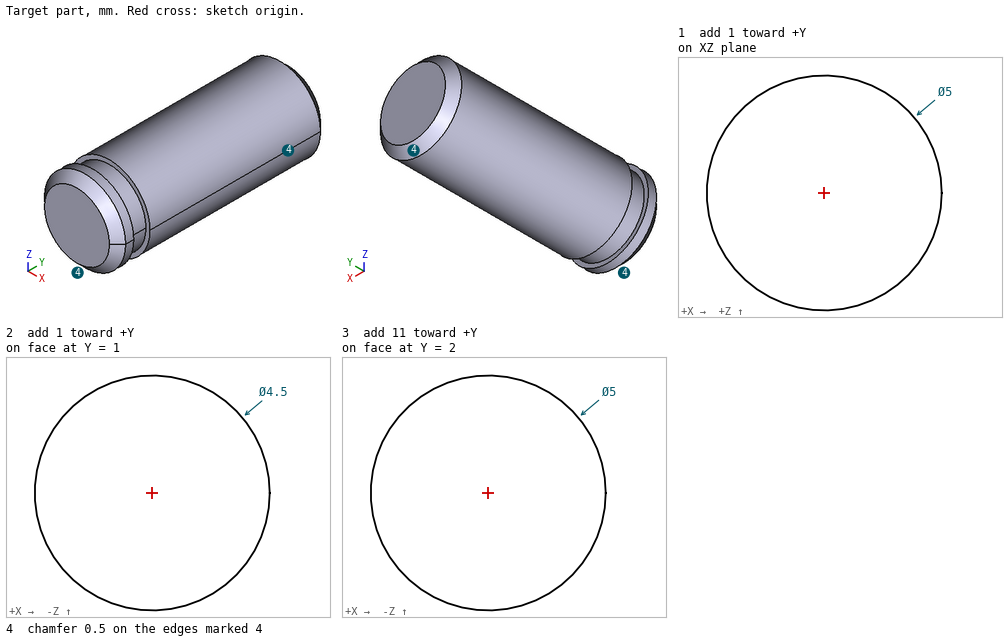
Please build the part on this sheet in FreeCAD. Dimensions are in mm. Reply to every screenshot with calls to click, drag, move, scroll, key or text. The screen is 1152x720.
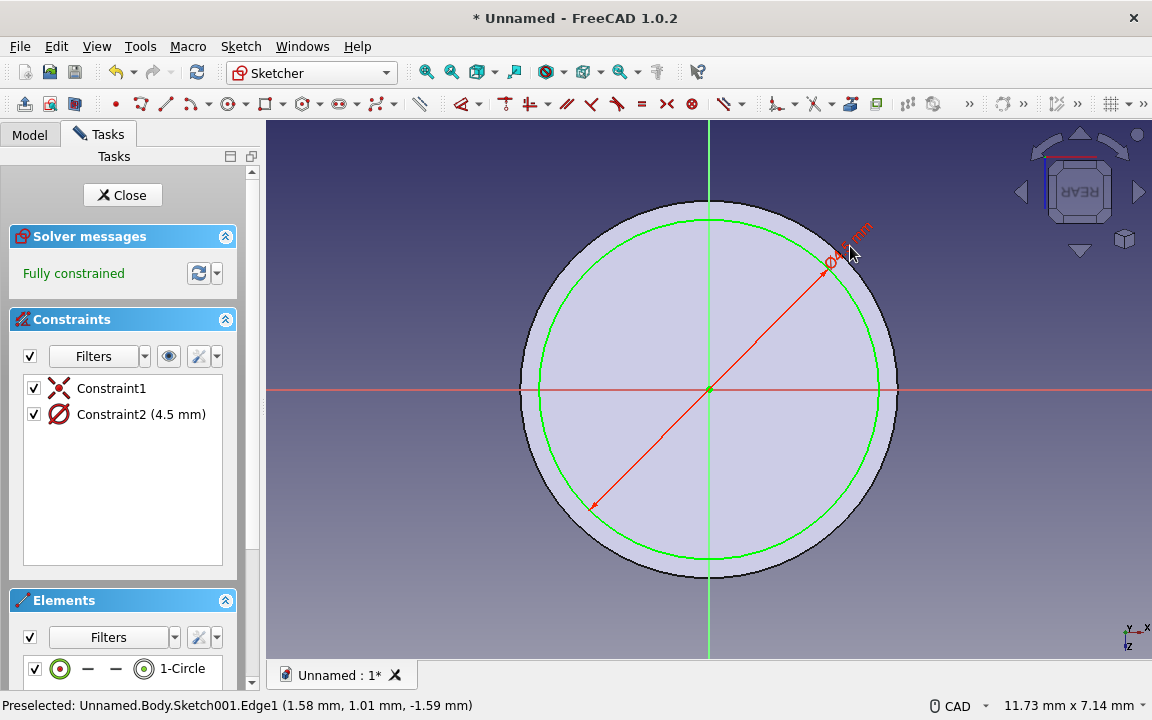
click(123, 195)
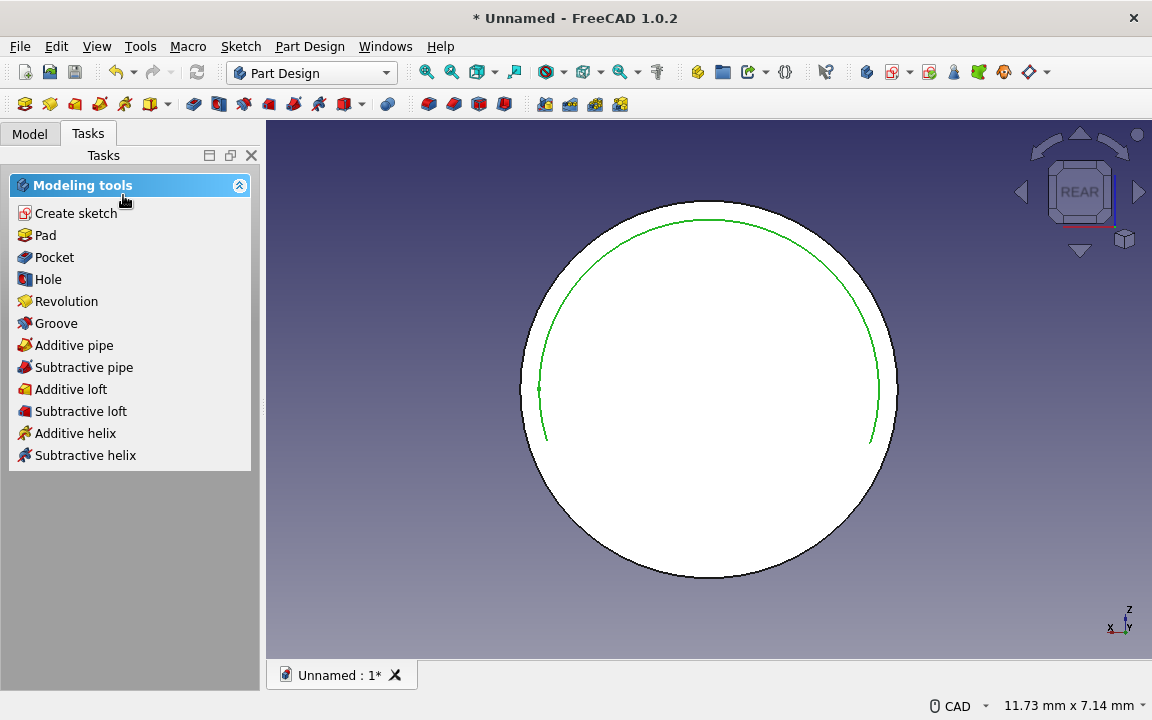
click(25, 104)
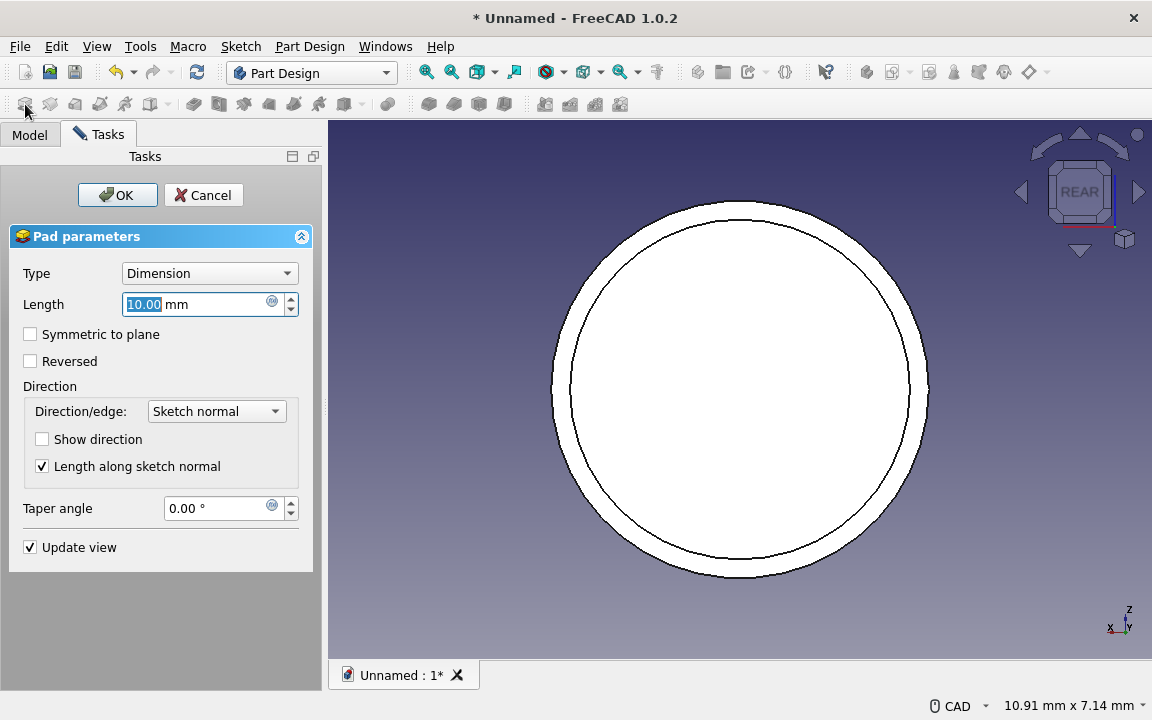
text(1)
key(Tab)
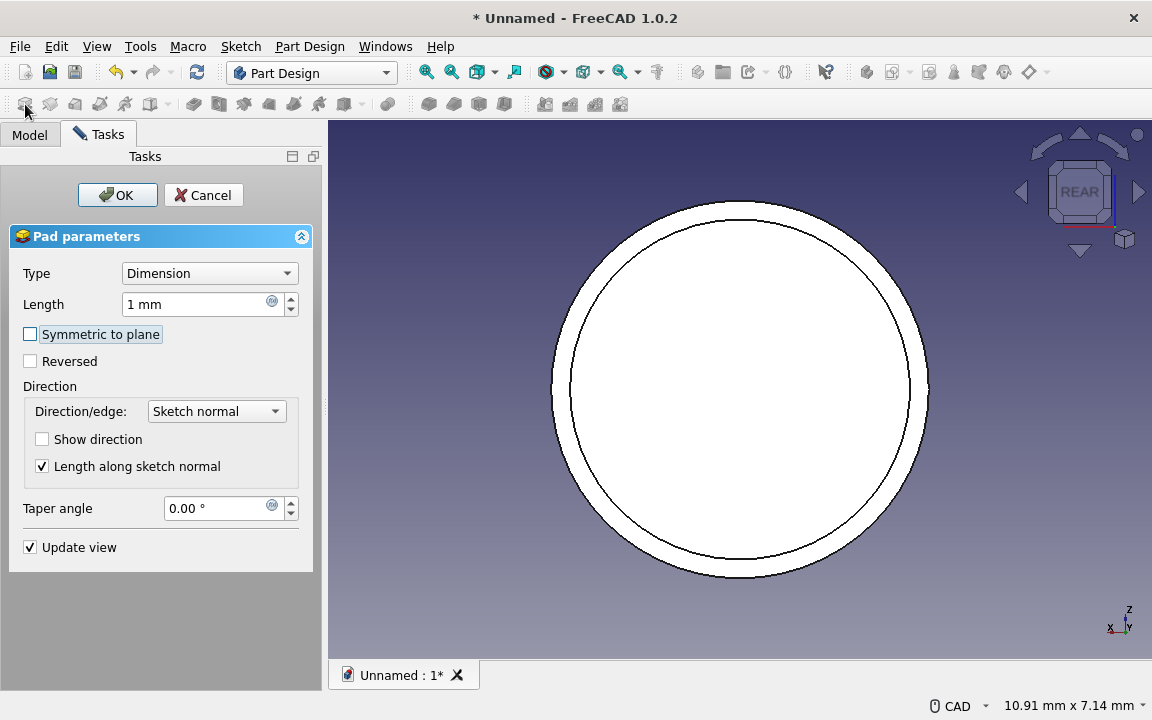
click(118, 195)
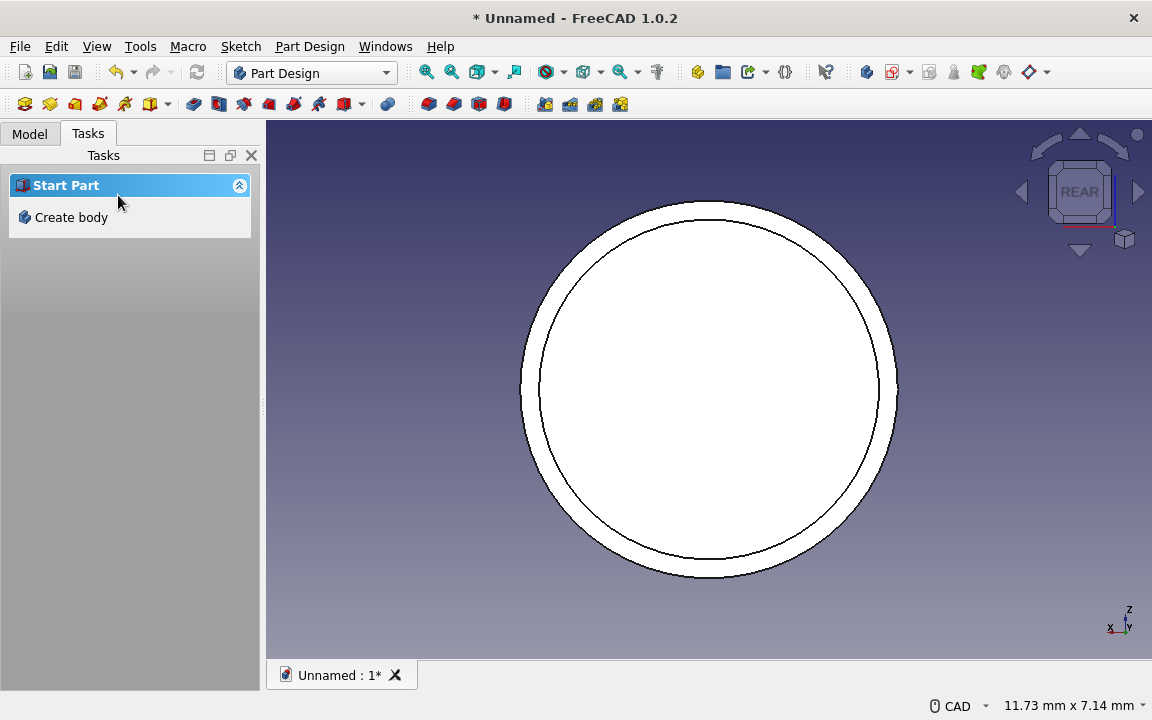
click(709, 388)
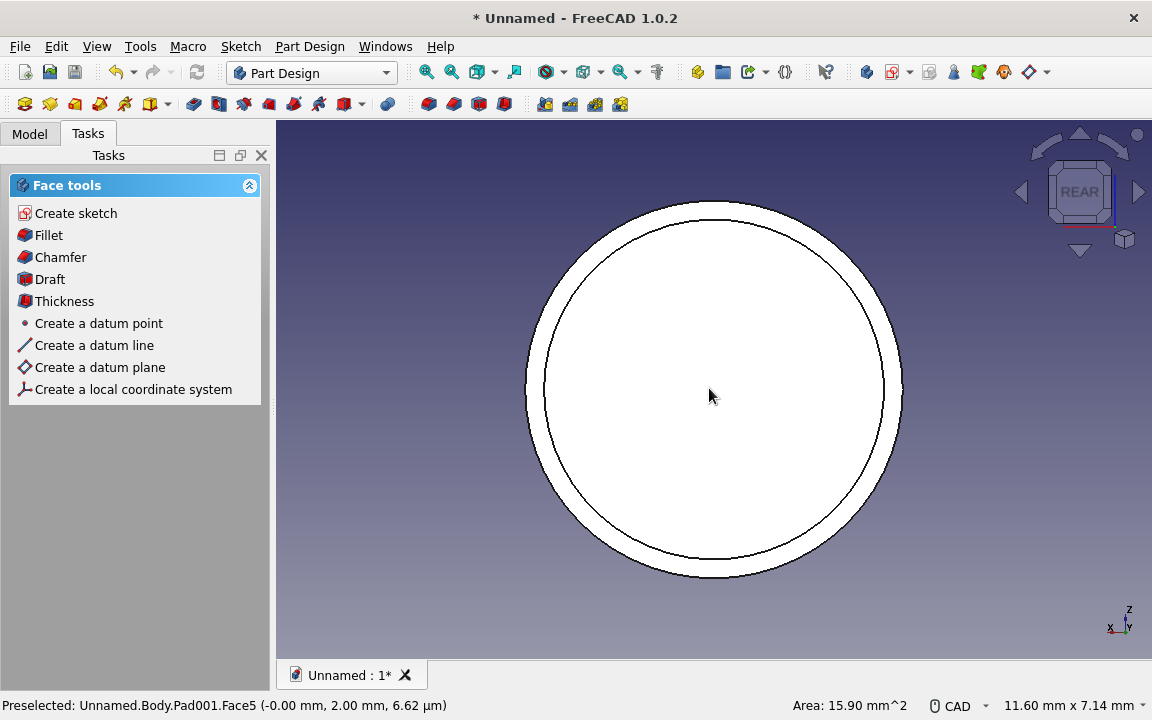
click(892, 72)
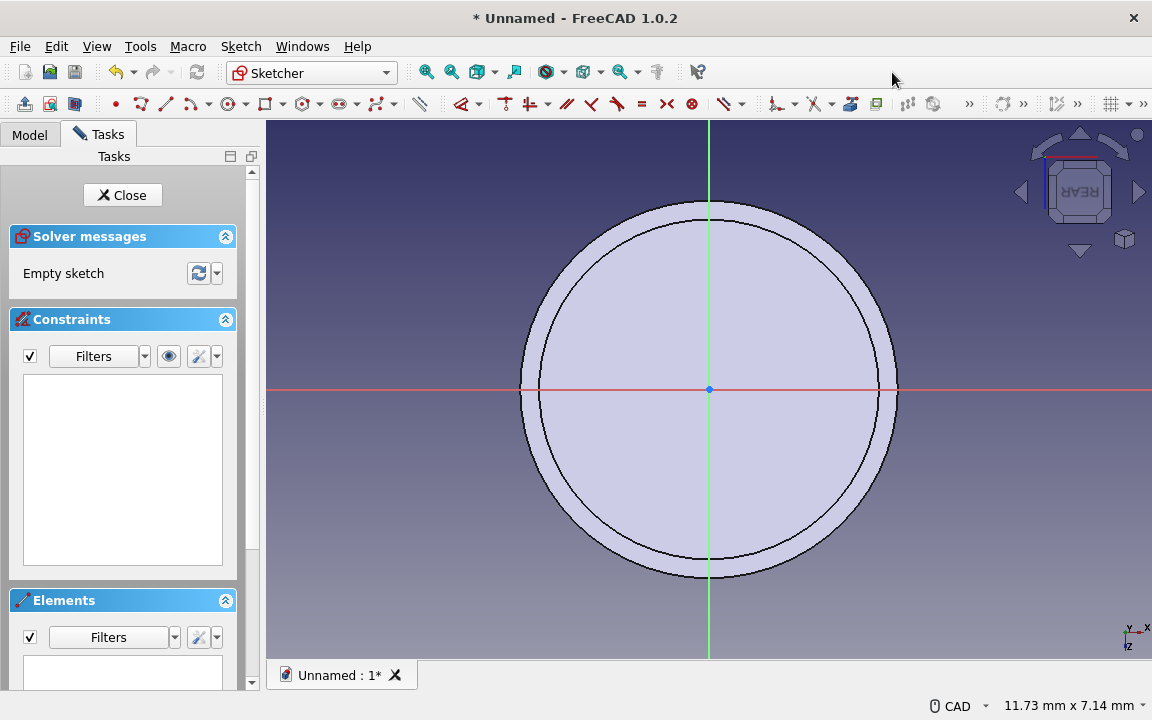
key(g)
key(c)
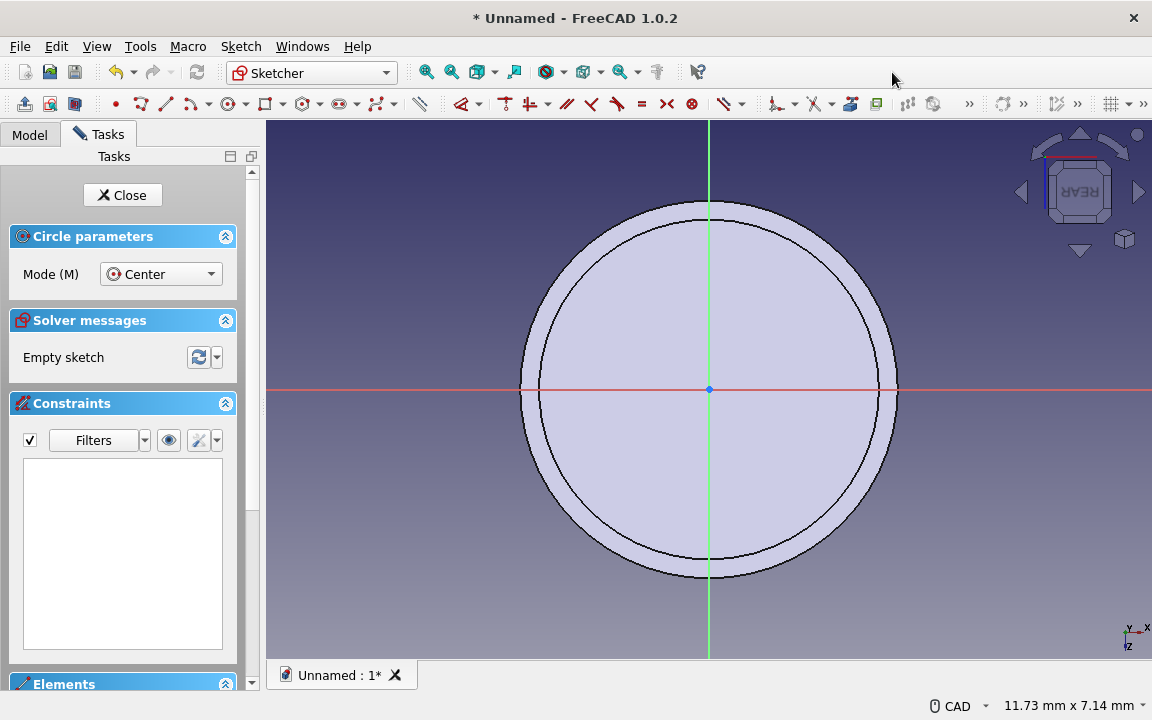
click(709, 389)
click(843, 256)
key(Escape)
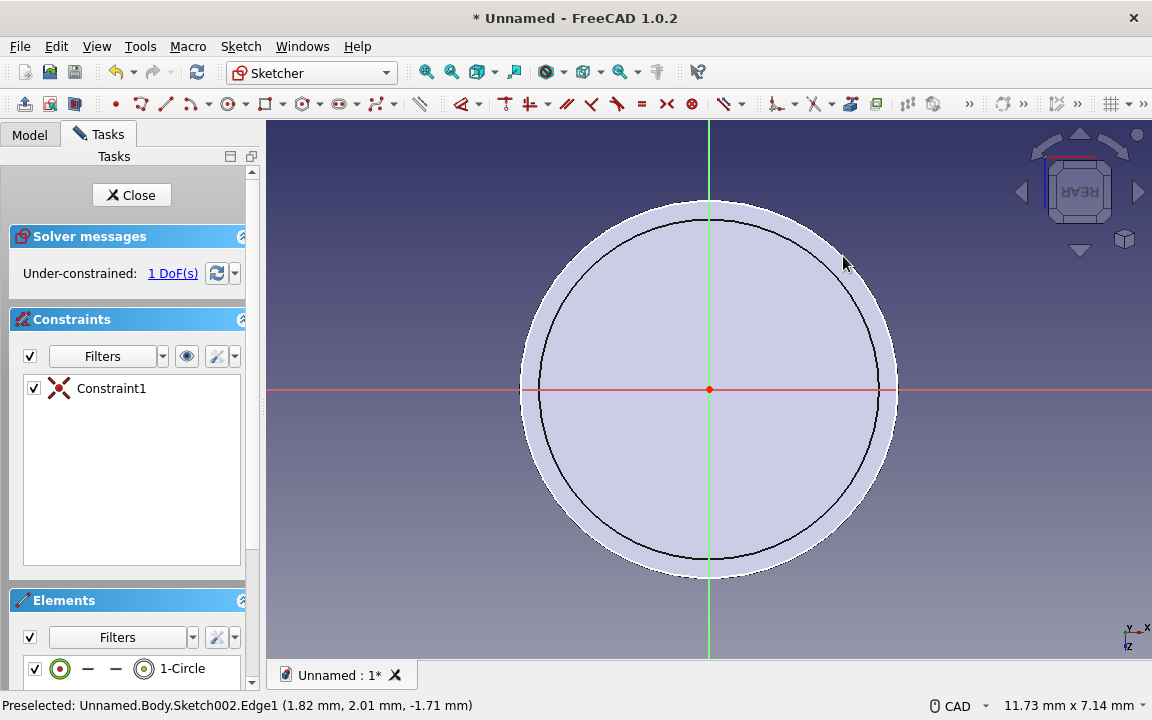
key(d)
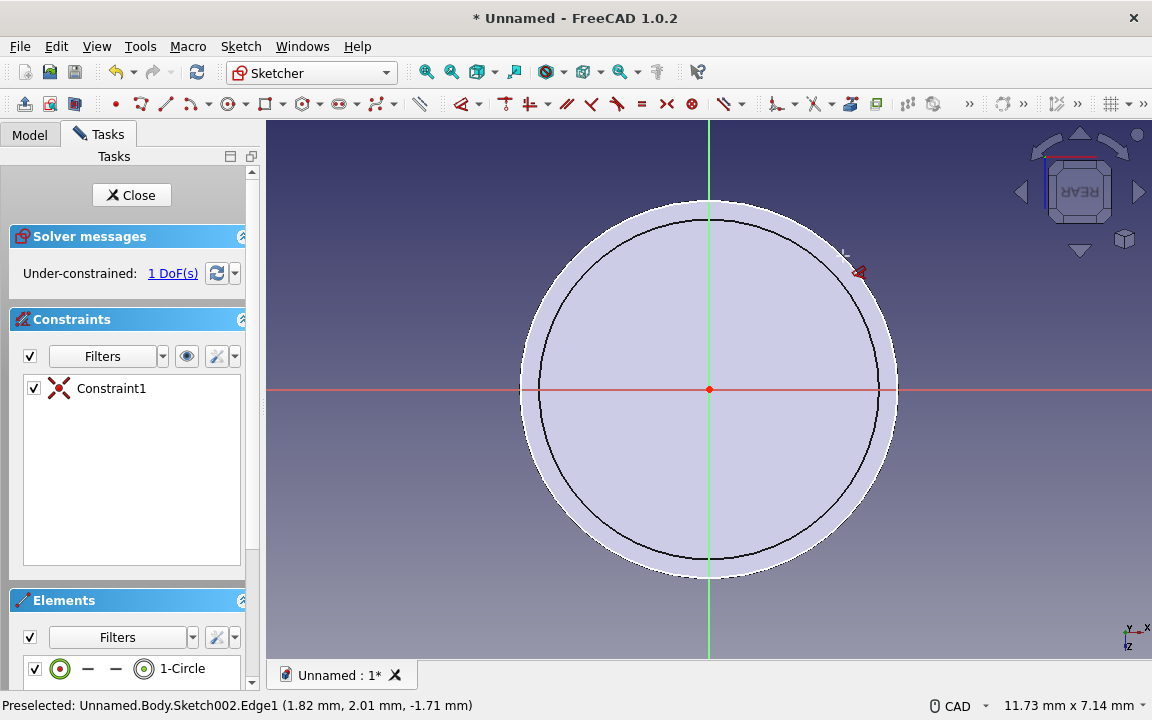
click(842, 256)
click(865, 233)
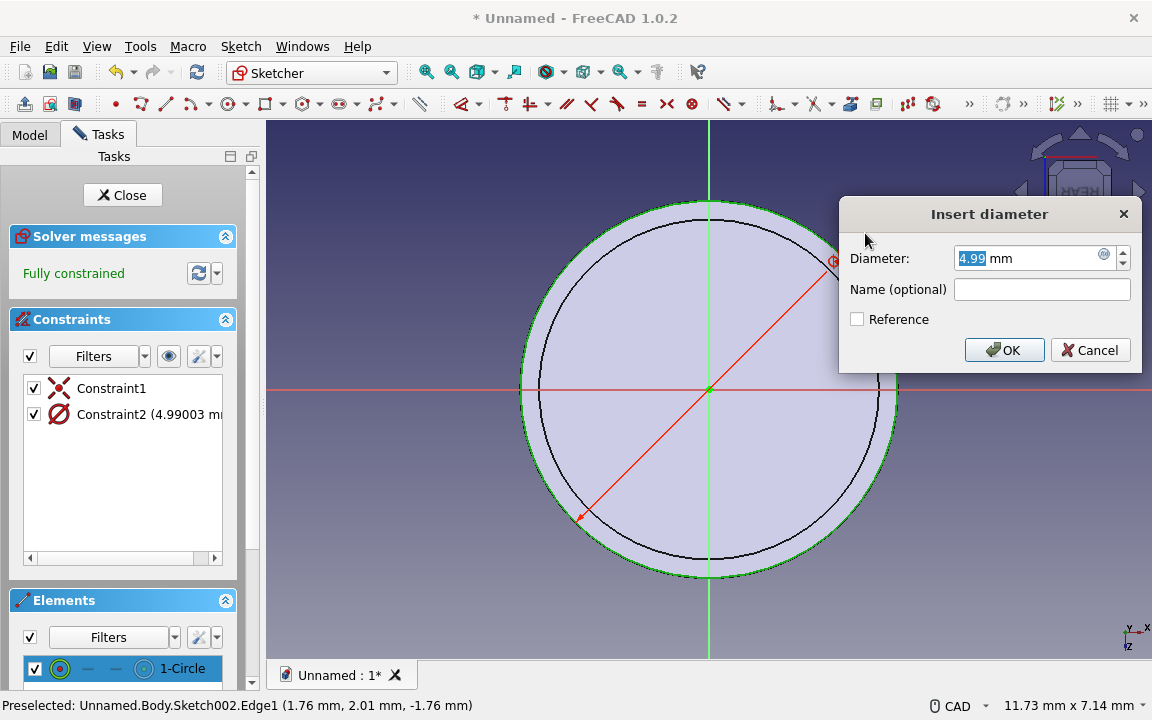
text(5)
key(Return)
key(Escape)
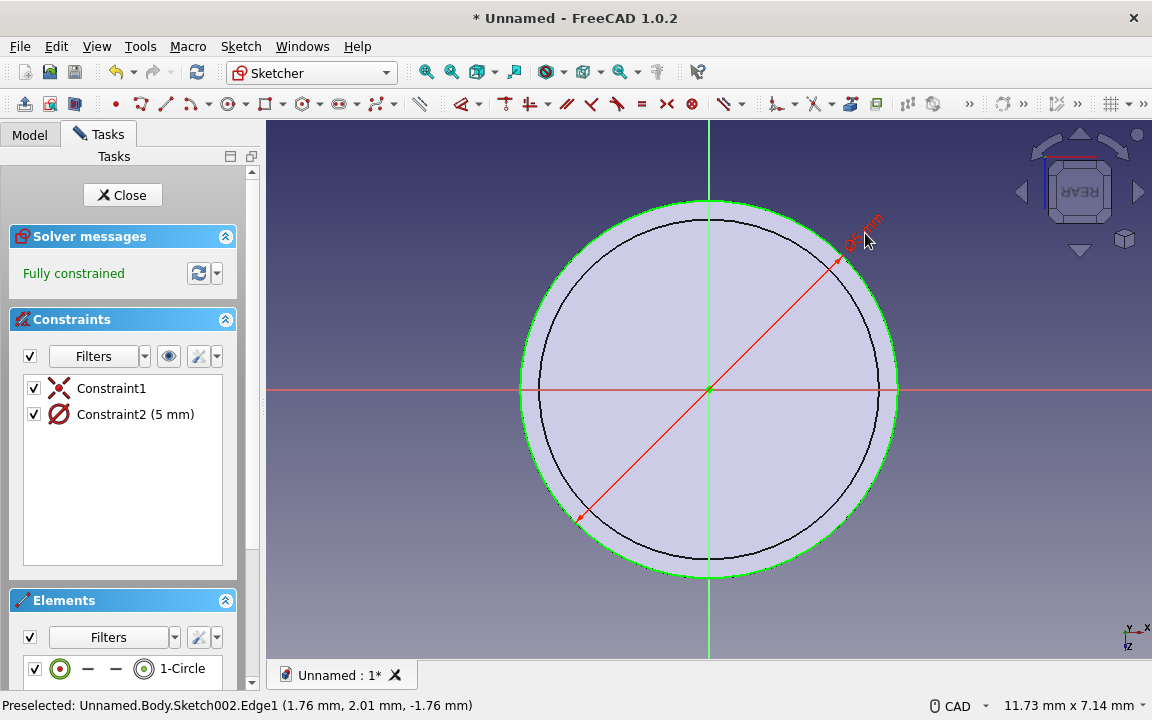
click(123, 195)